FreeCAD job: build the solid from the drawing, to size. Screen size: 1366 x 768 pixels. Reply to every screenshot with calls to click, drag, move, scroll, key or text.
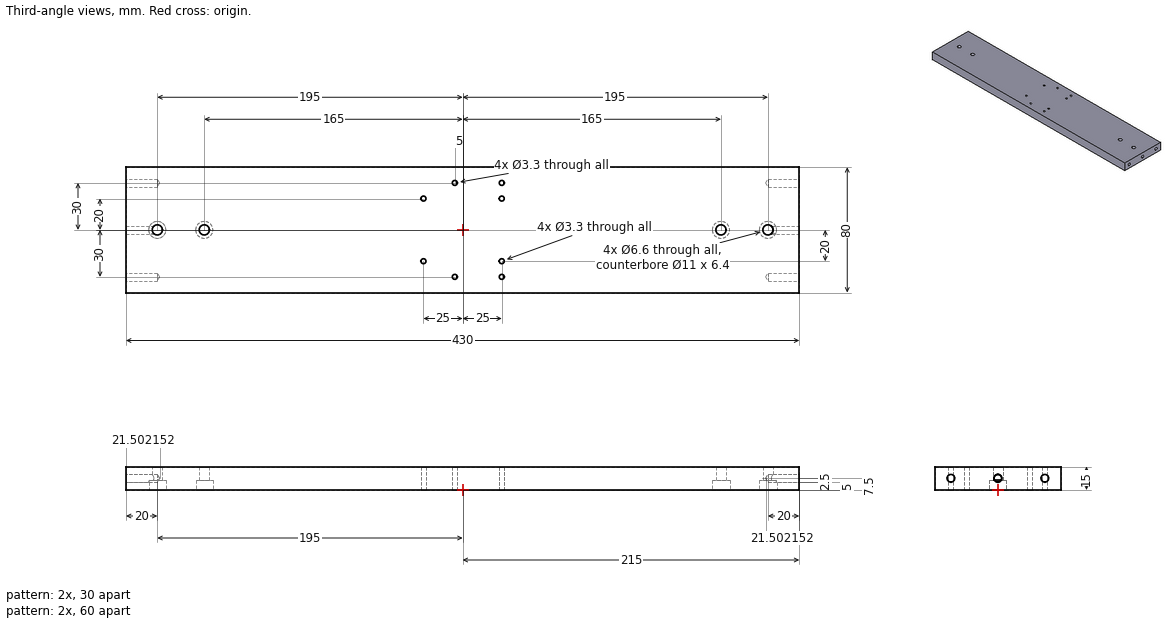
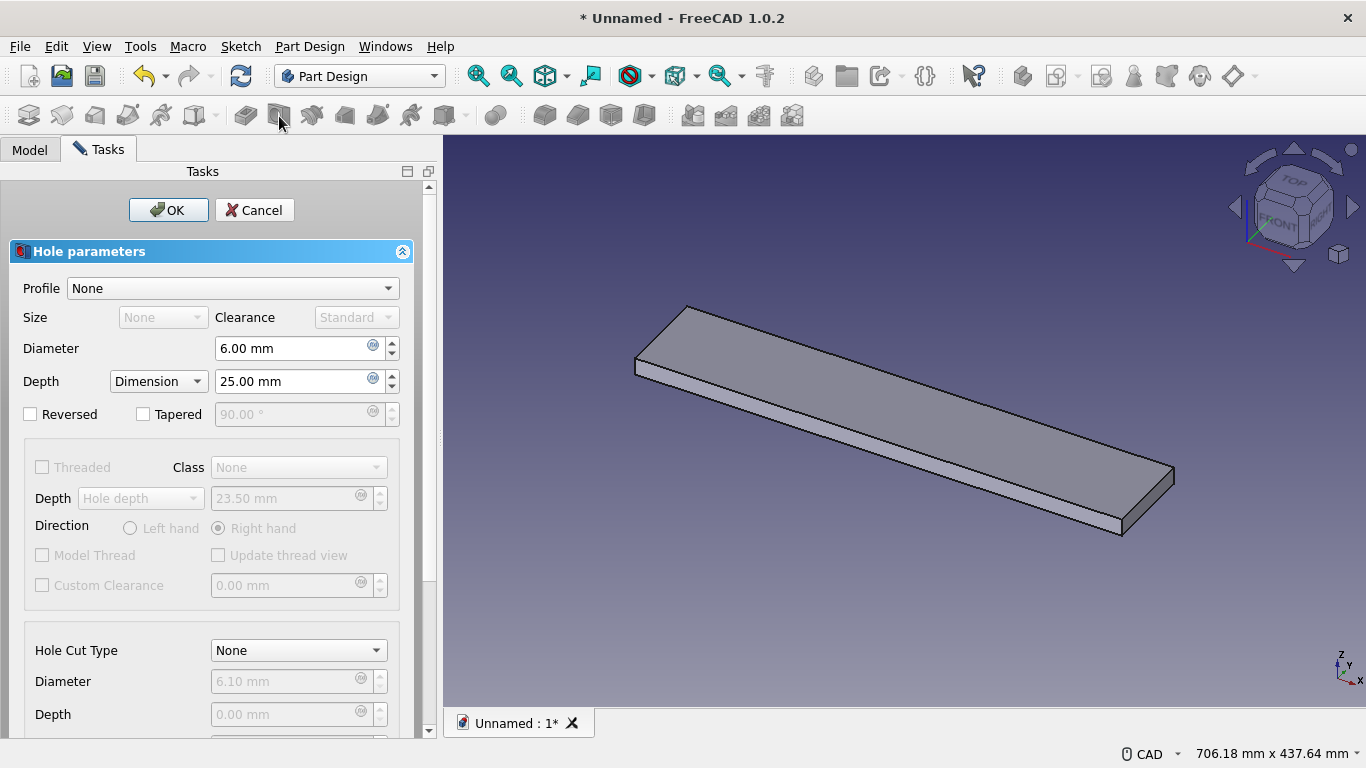
triple_click(300, 348)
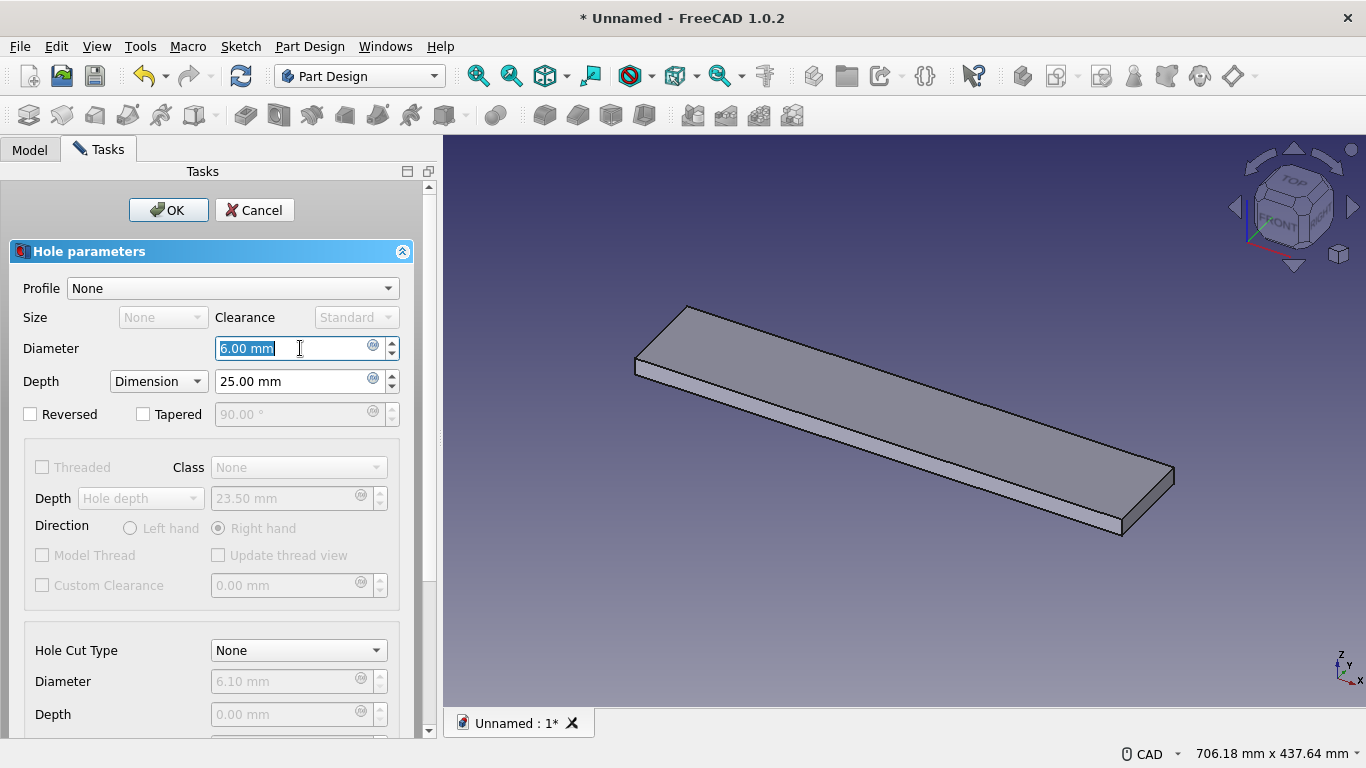
text(3.3)
key(Tab)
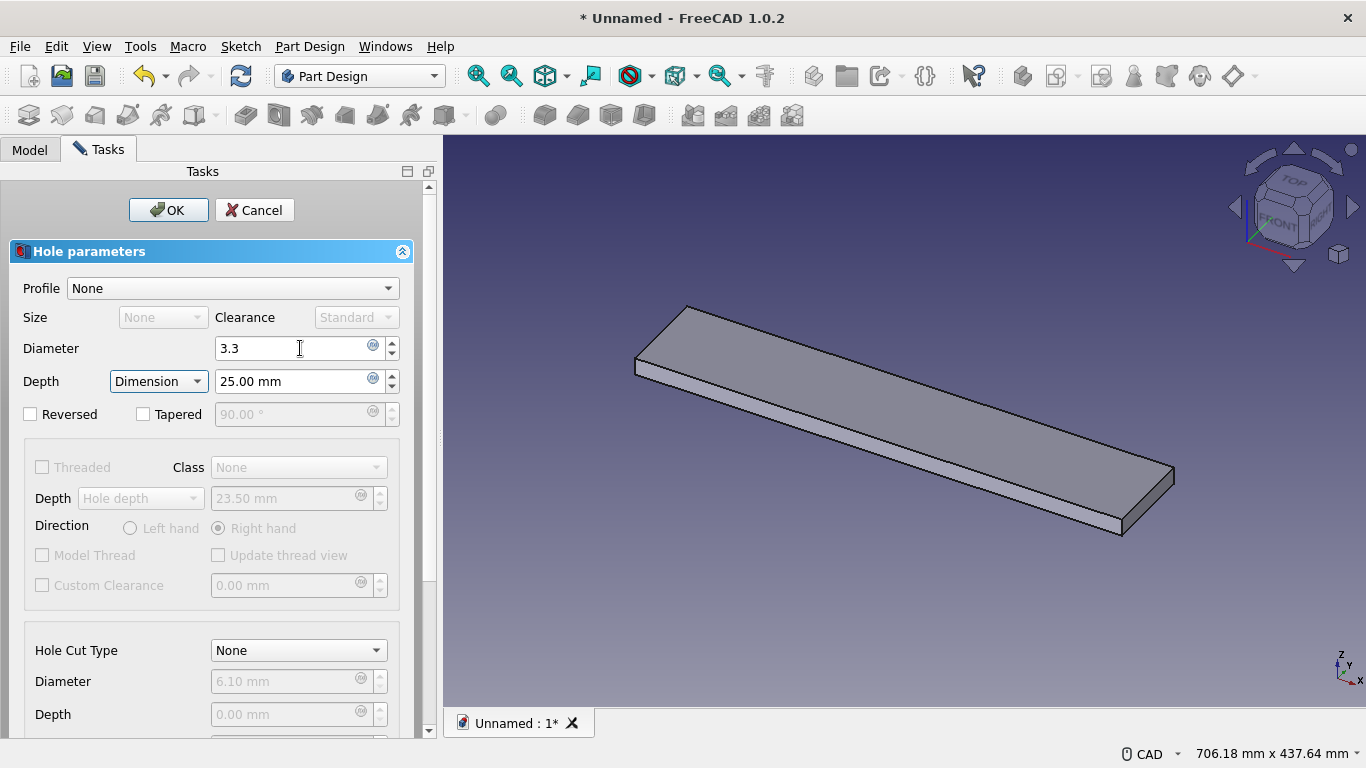
click(160, 382)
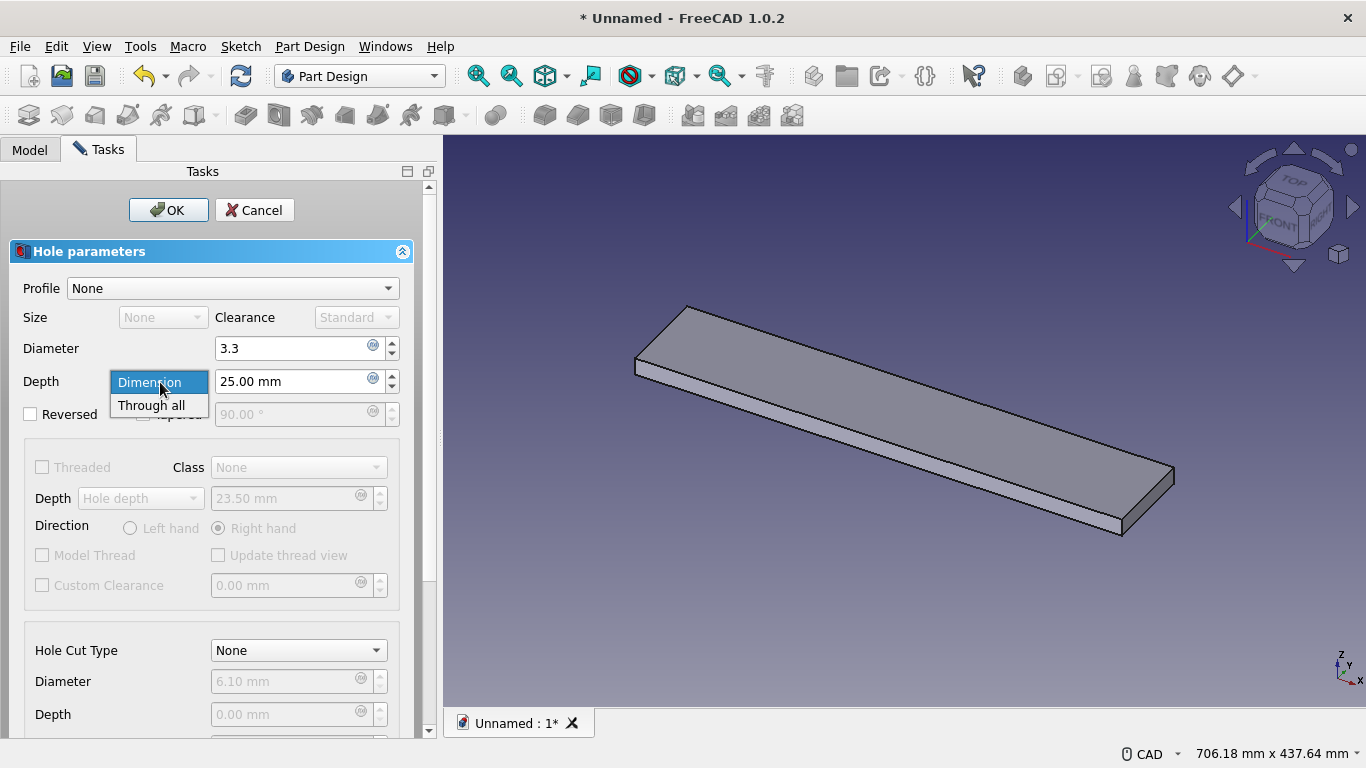
click(158, 406)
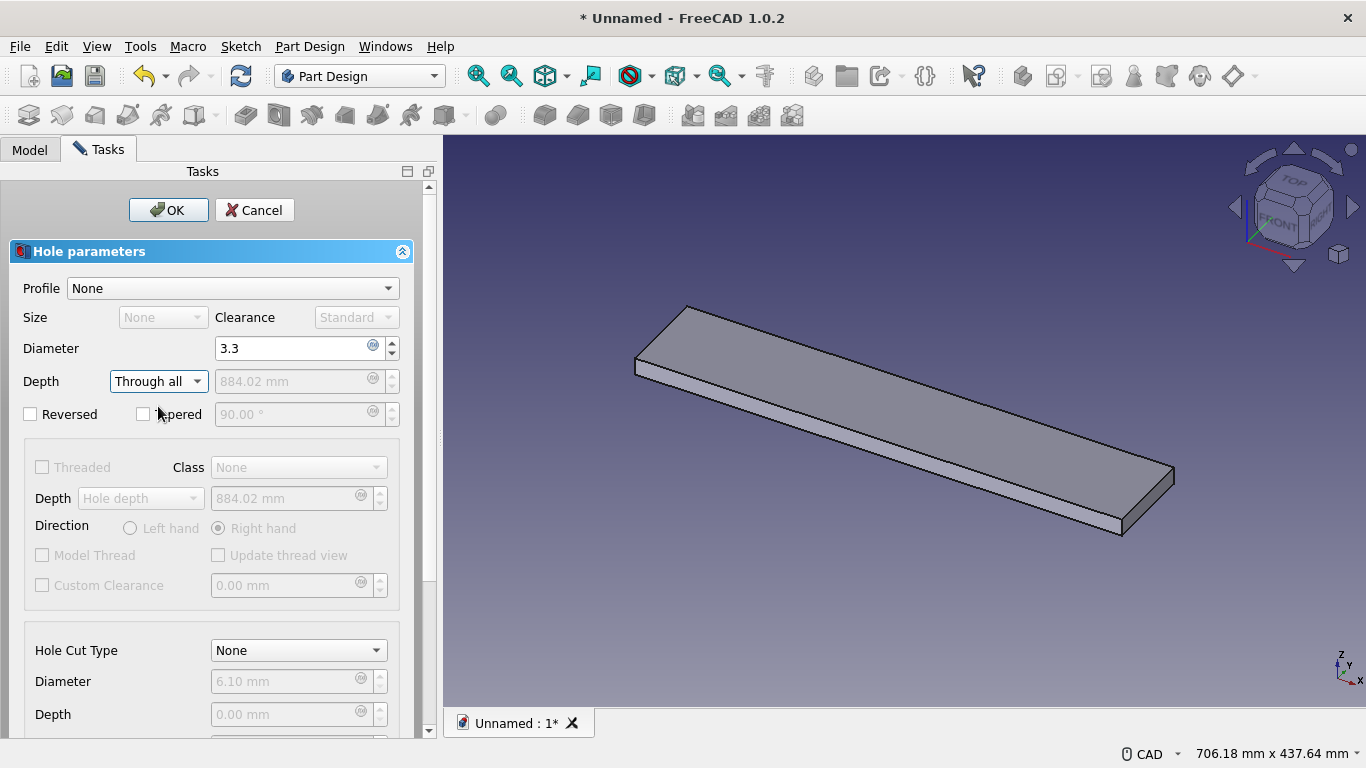
click(31, 414)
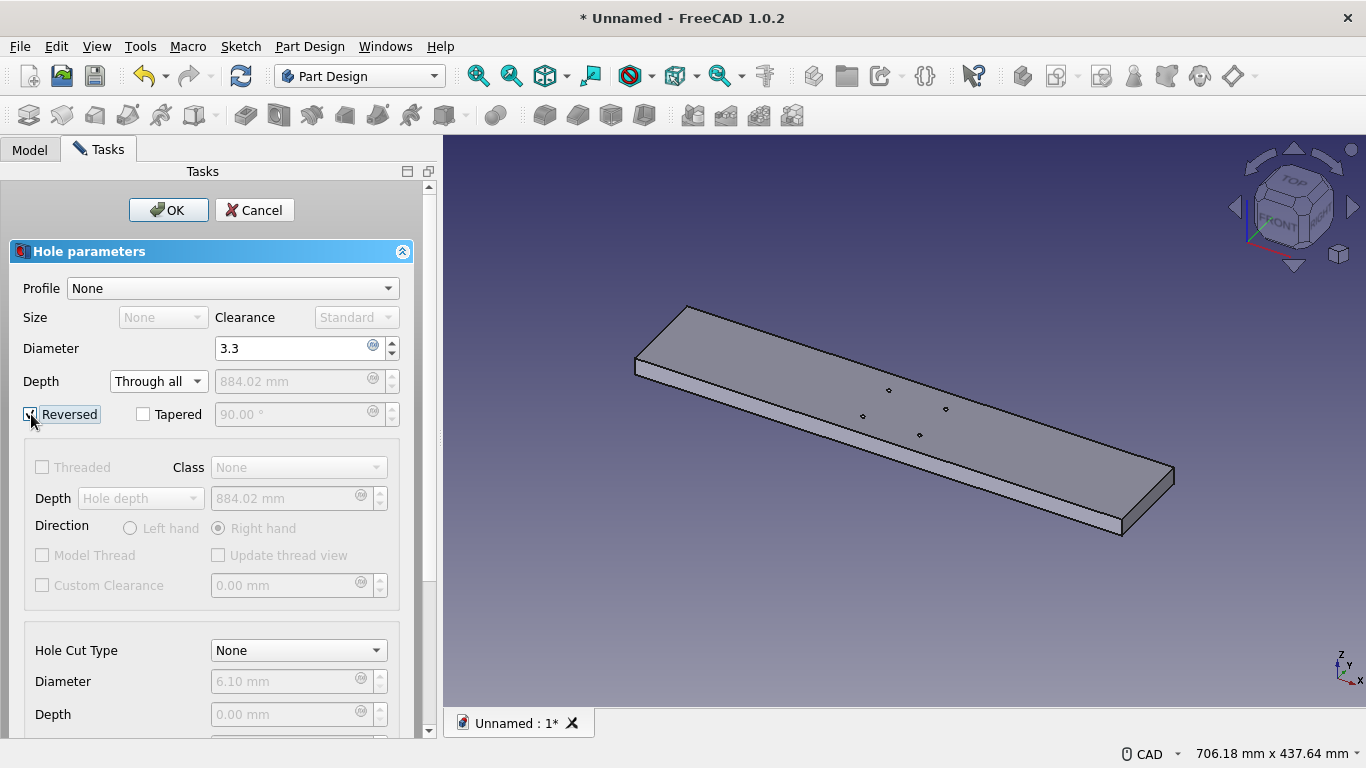
click(169, 210)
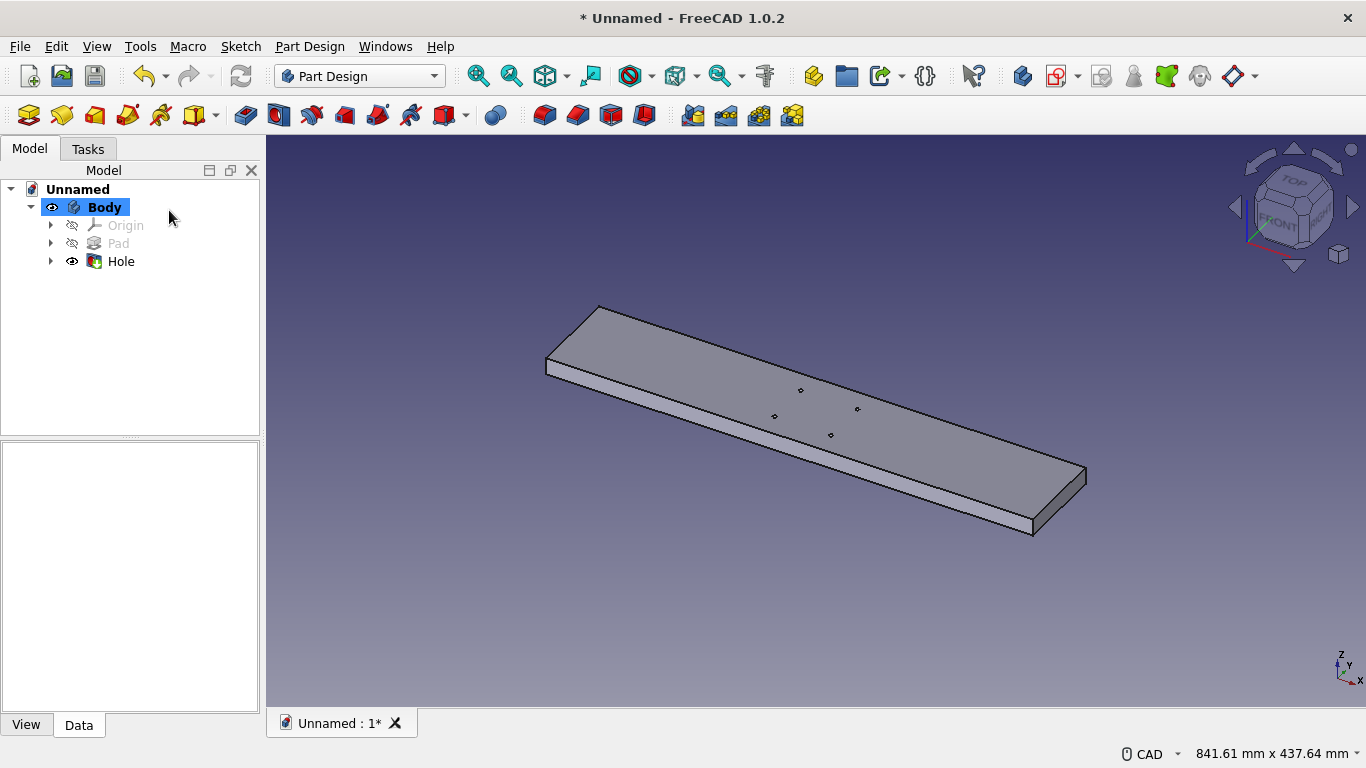
key(5)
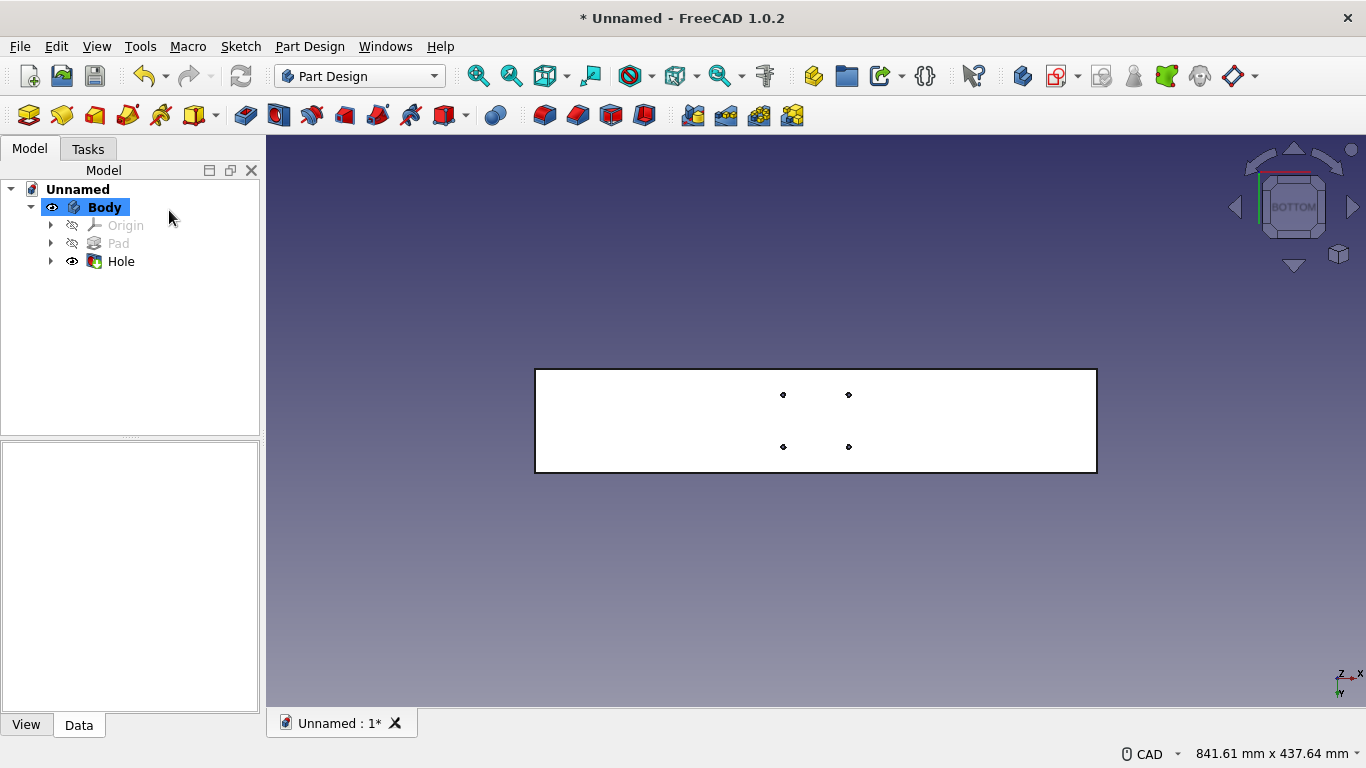
click(977, 420)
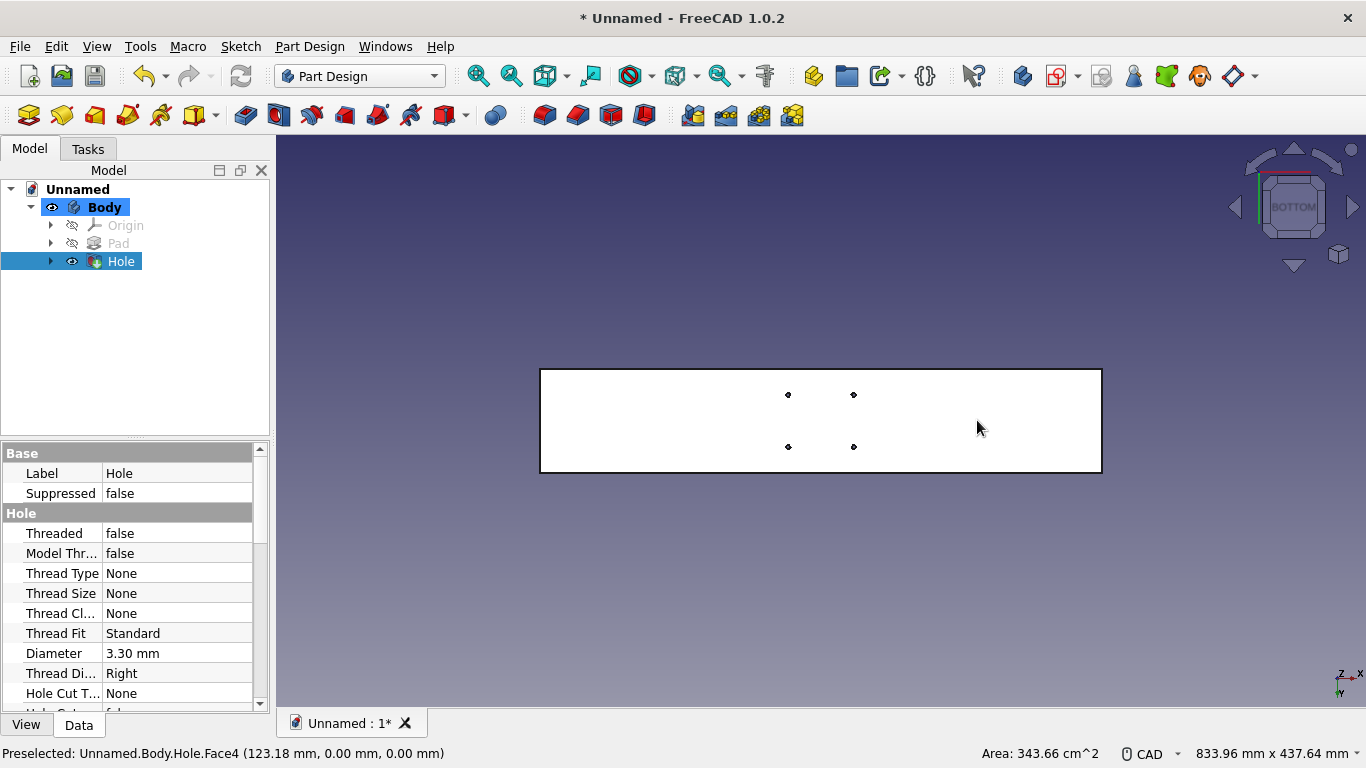
click(1056, 76)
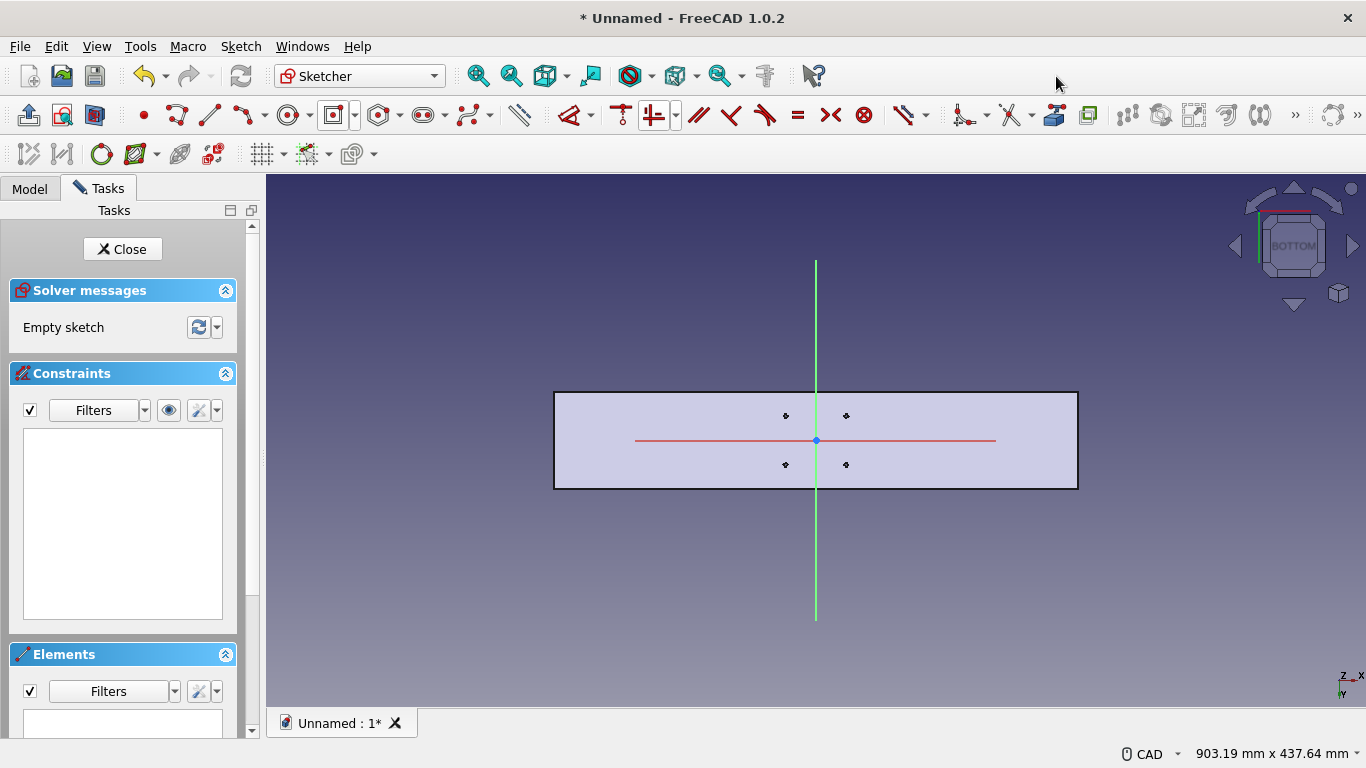
scroll(855, 440, up, 7)